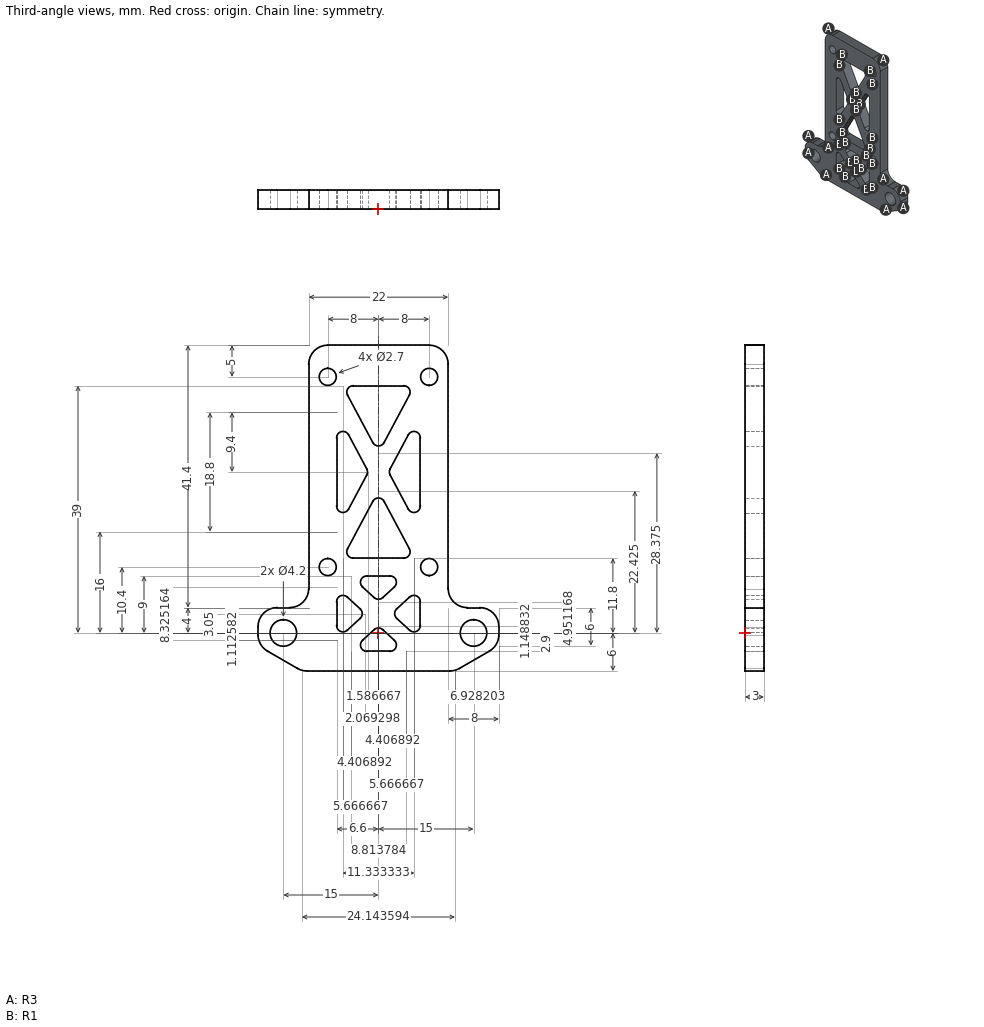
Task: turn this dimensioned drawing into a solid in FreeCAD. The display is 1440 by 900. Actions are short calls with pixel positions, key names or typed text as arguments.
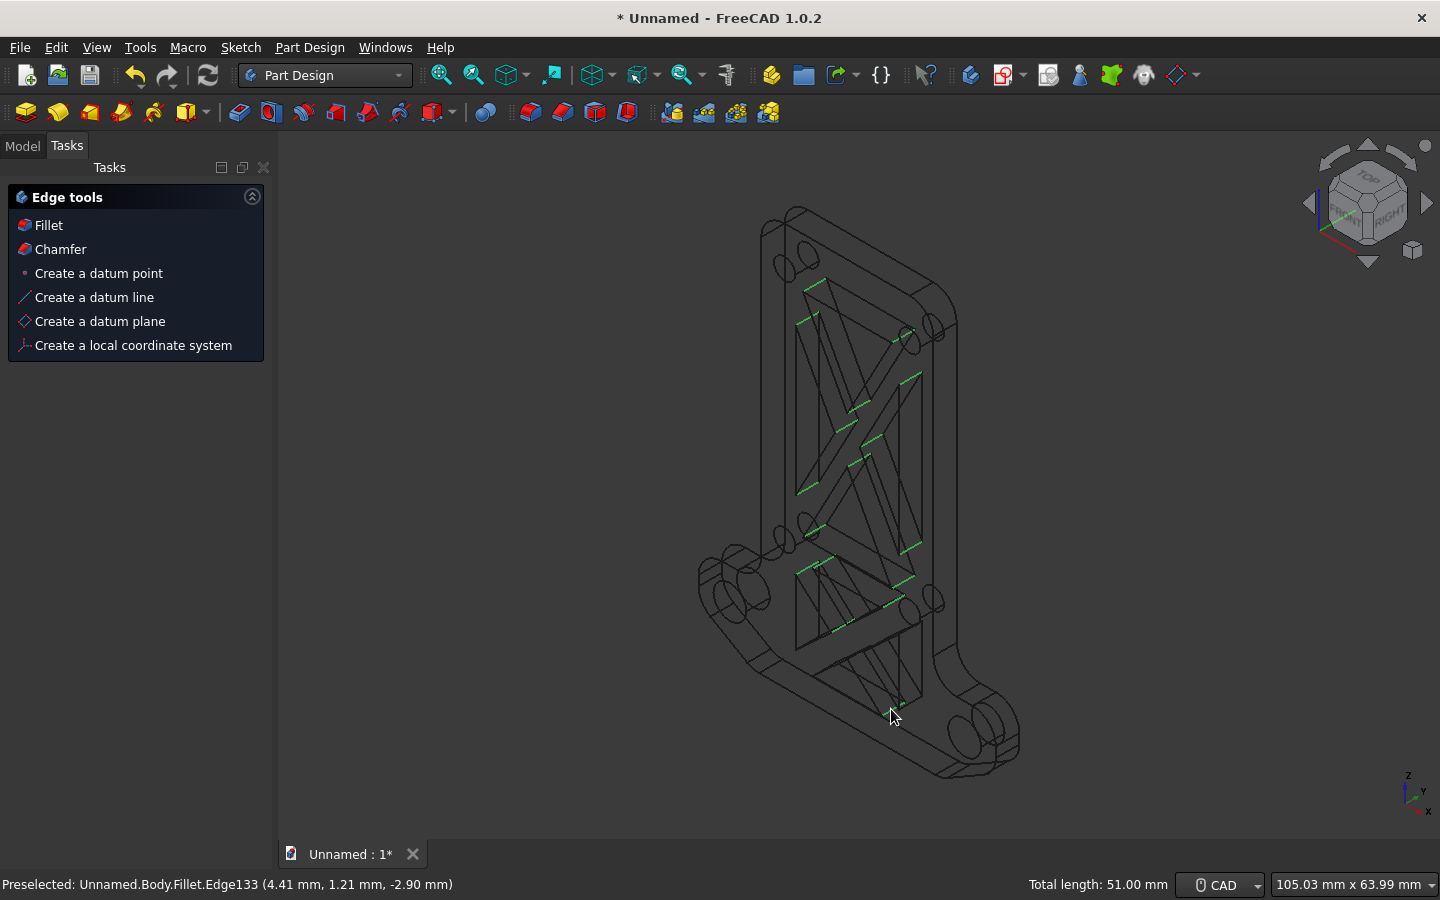
click(857, 653, ctrl)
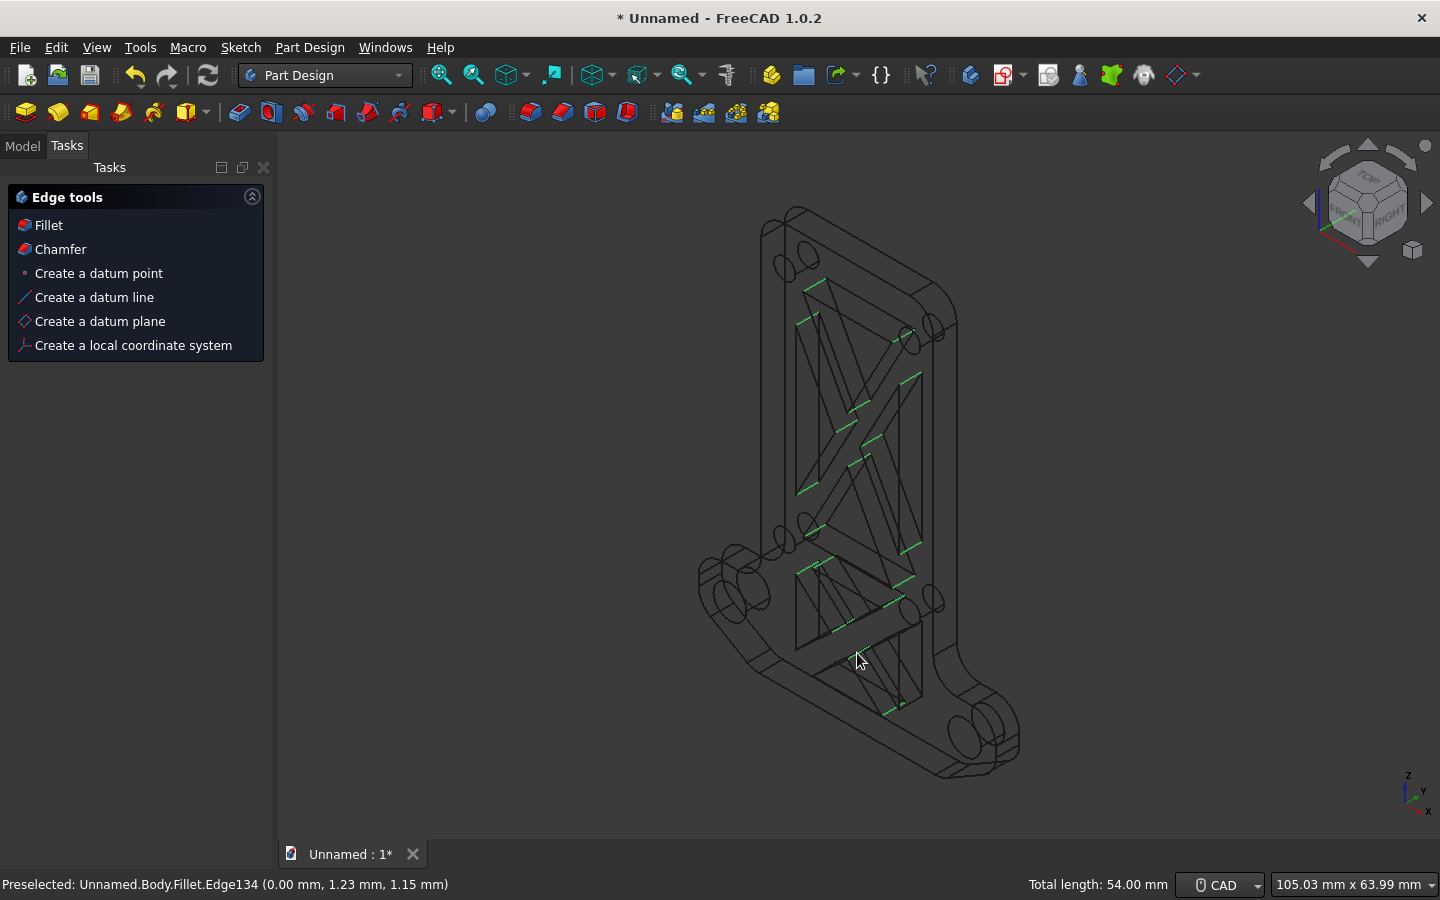
click(911, 702, ctrl)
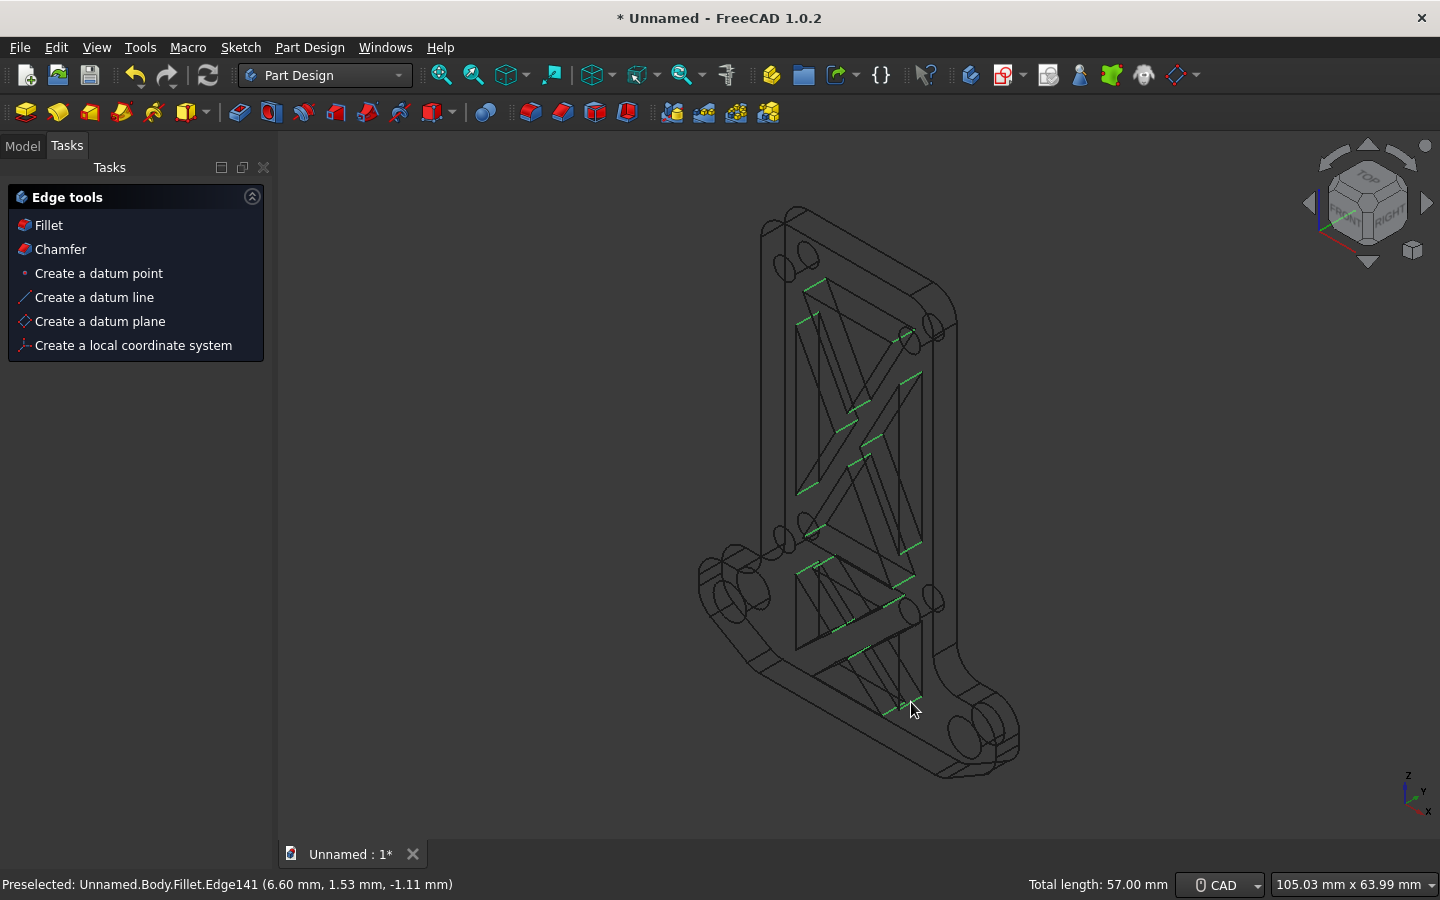
click(906, 629, ctrl)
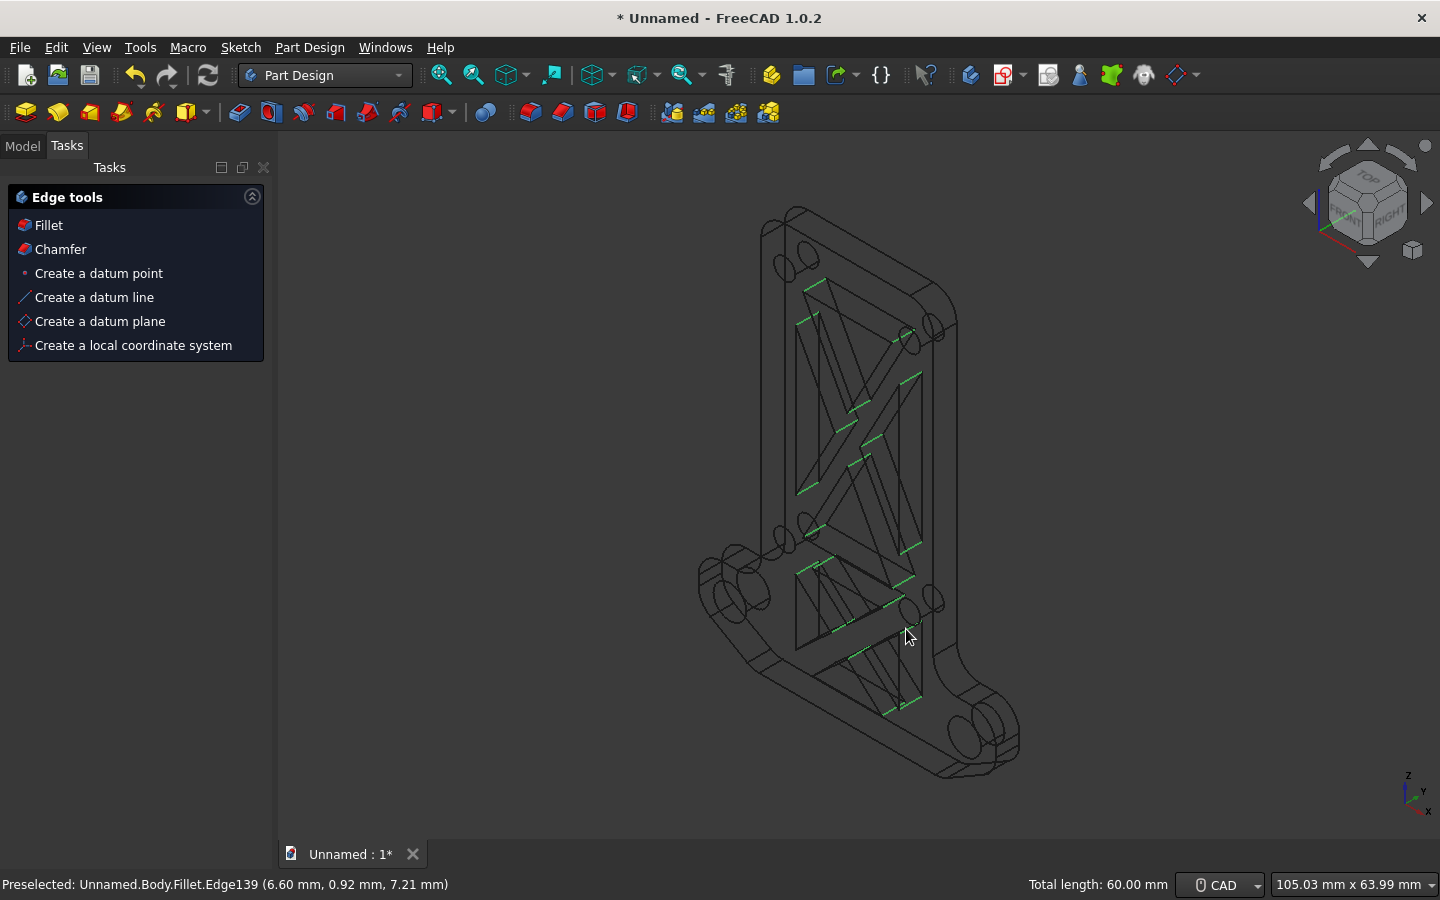
scroll(807, 642, up, 6)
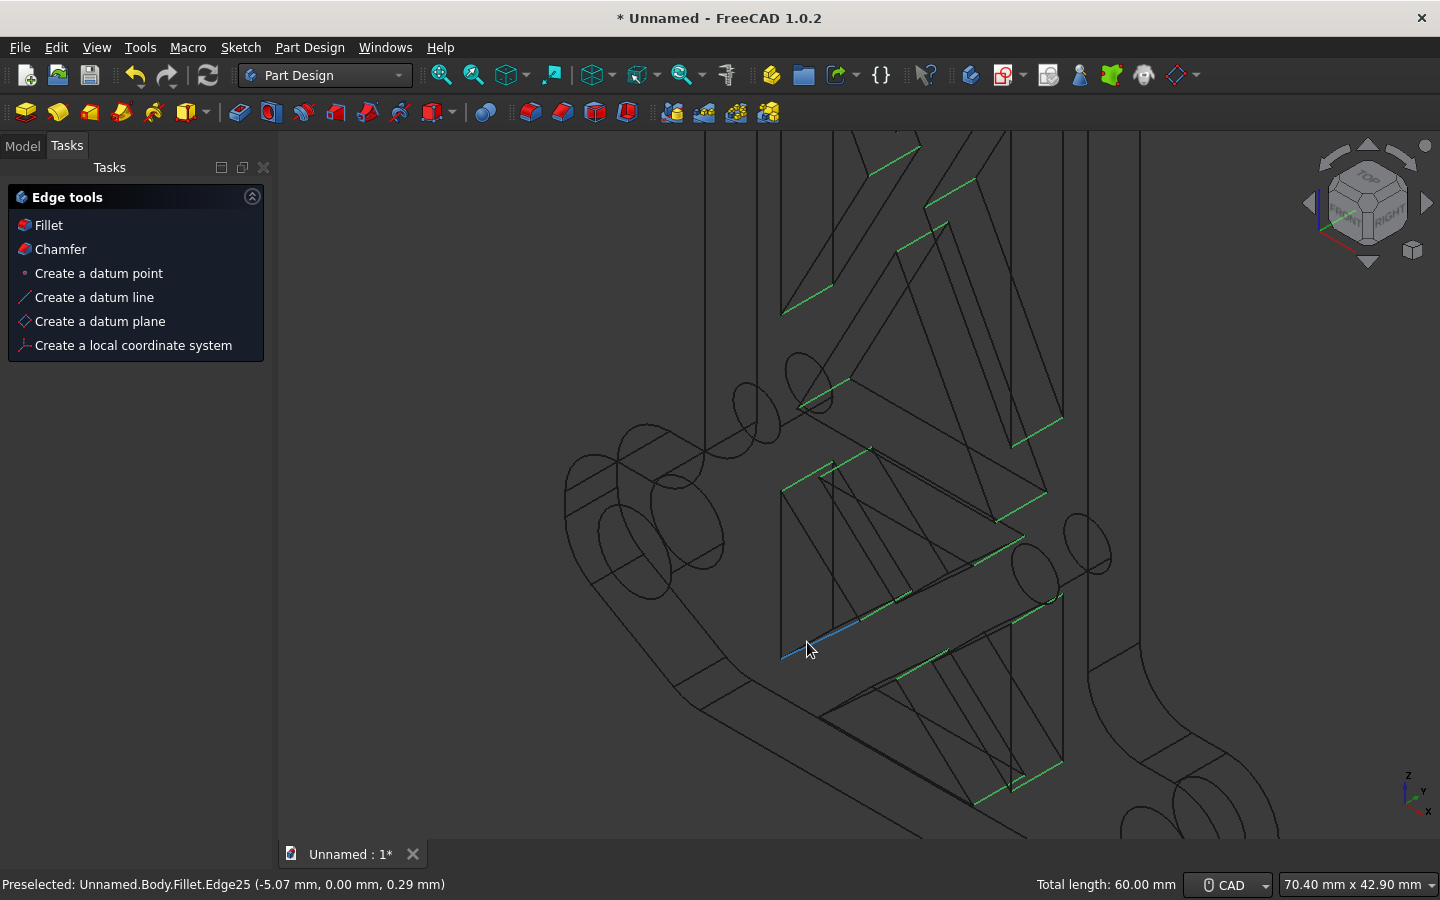
click(442, 76)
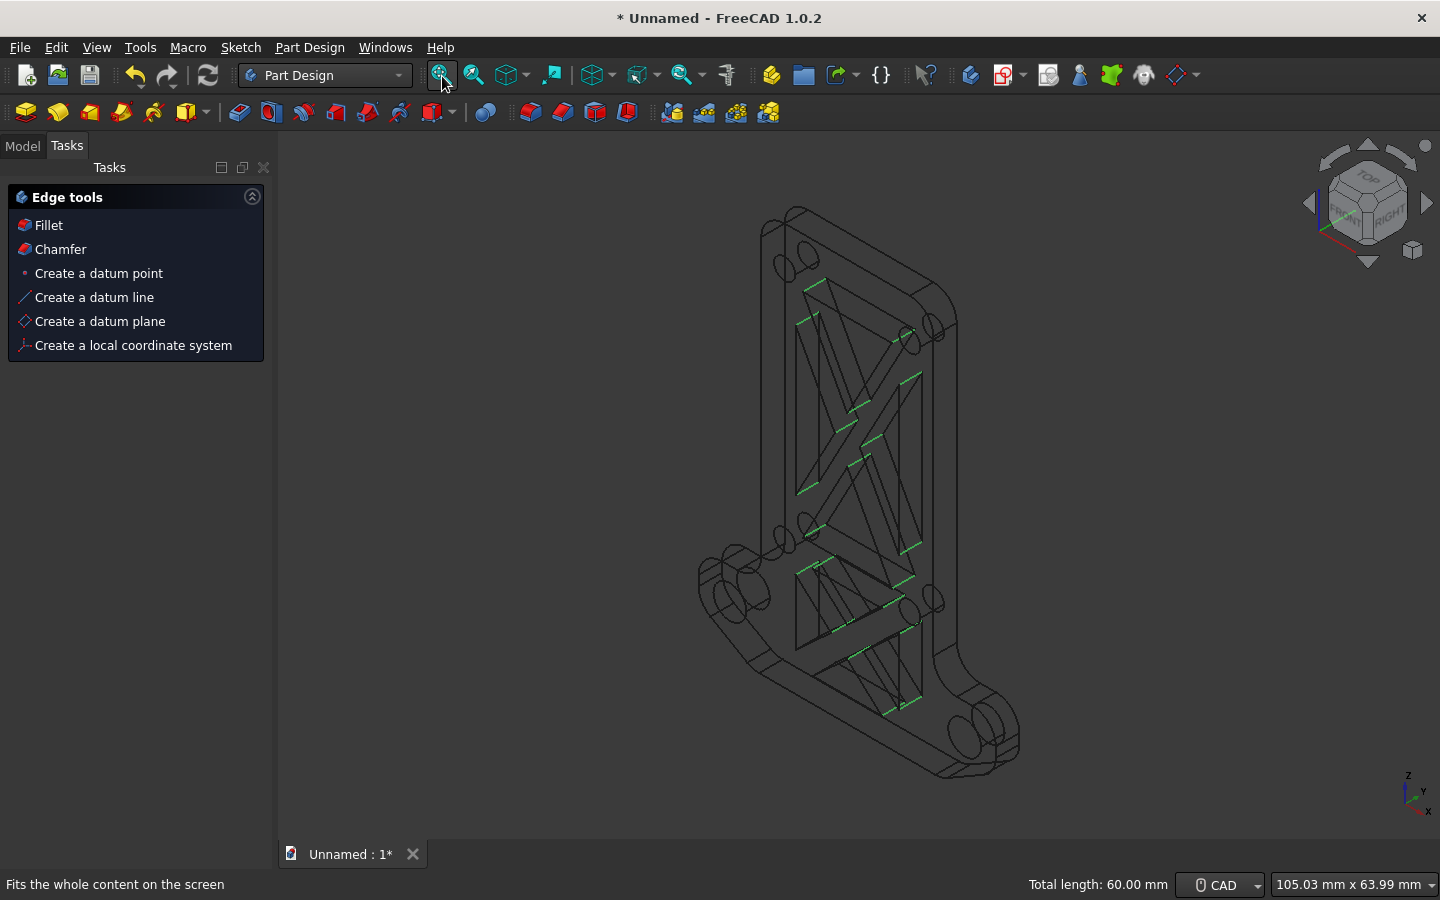
key(2)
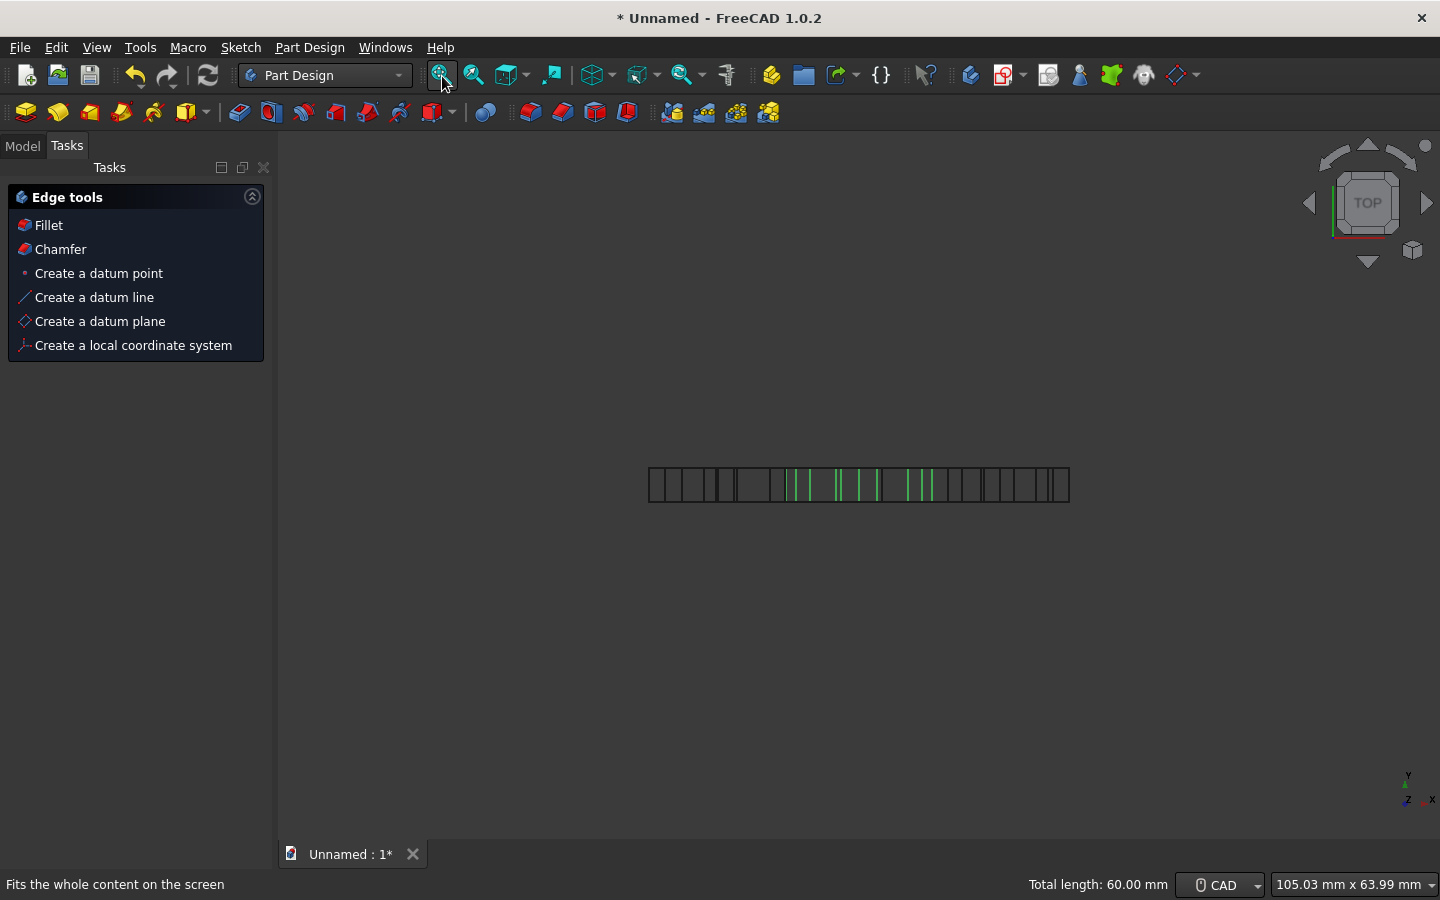
click(442, 76)